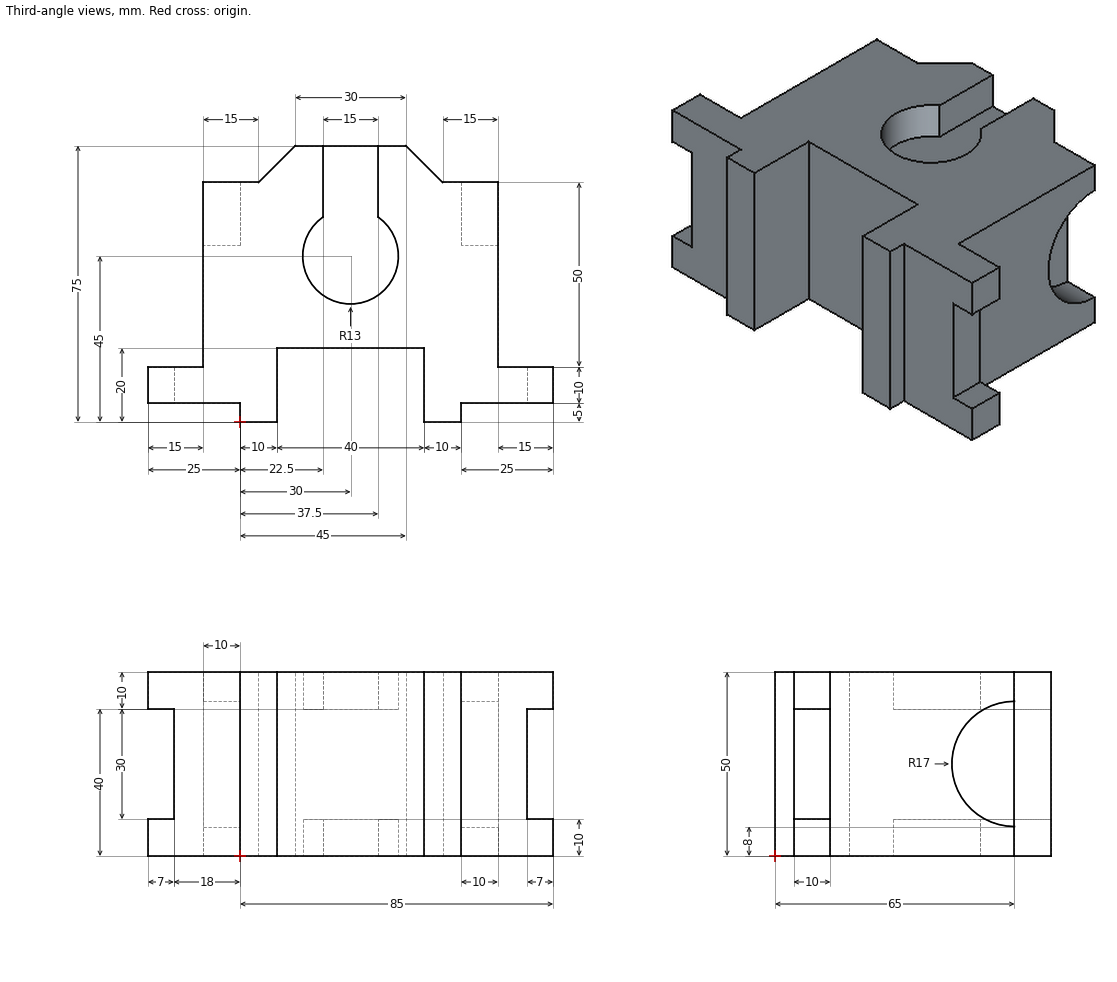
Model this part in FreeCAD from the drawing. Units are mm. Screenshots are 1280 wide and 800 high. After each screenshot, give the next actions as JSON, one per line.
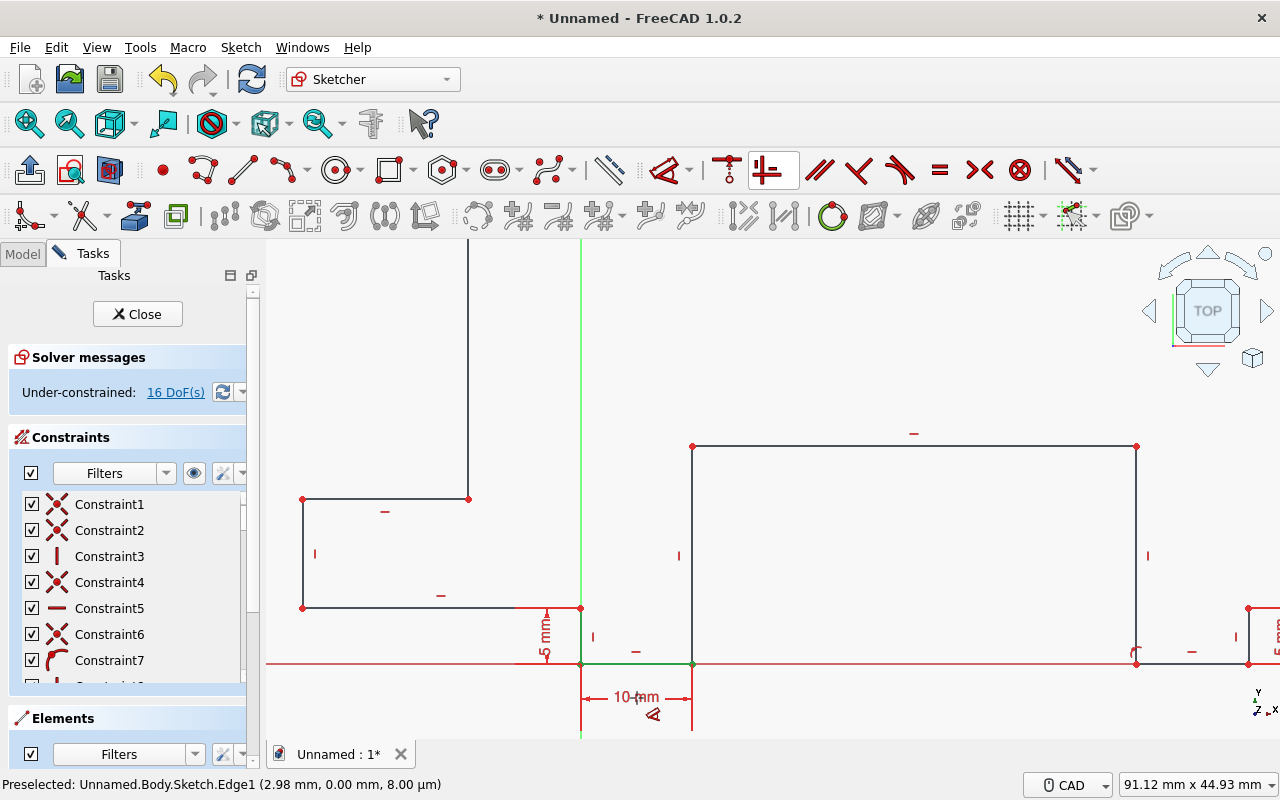
{"action": "left_click", "coordinate": [692, 599]}
{"action": "left_click", "coordinate": [658, 555]}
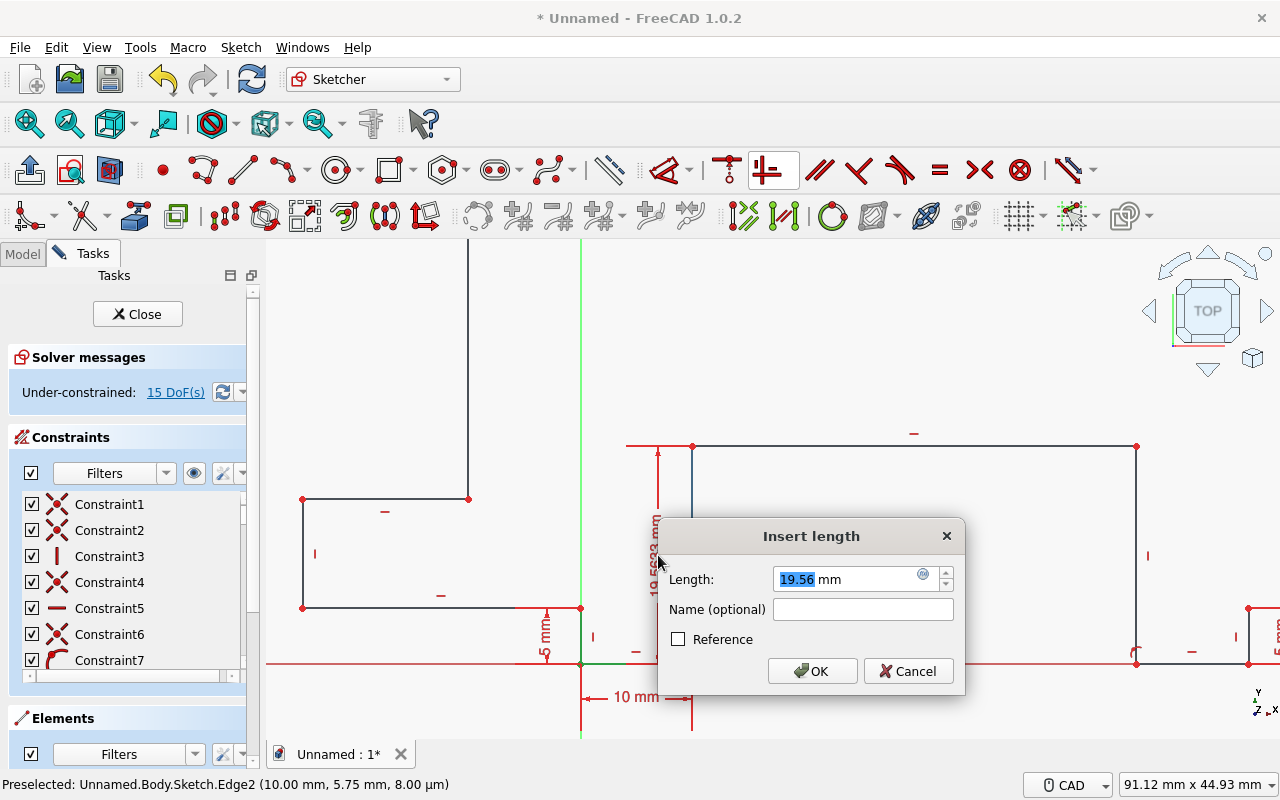
{"action": "type", "text": "20"}
{"action": "key", "text": "Return"}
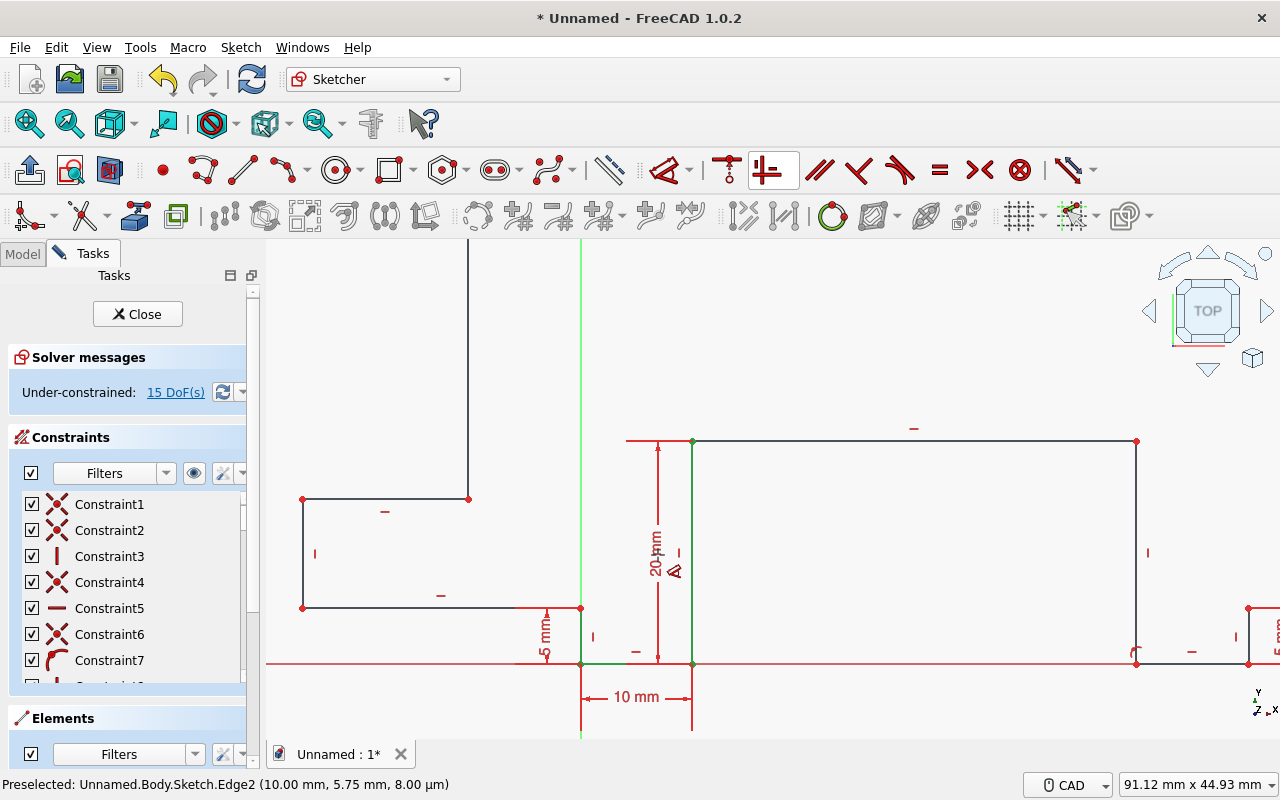
{"action": "left_click", "coordinate": [825, 441]}
{"action": "left_click", "coordinate": [904, 475]}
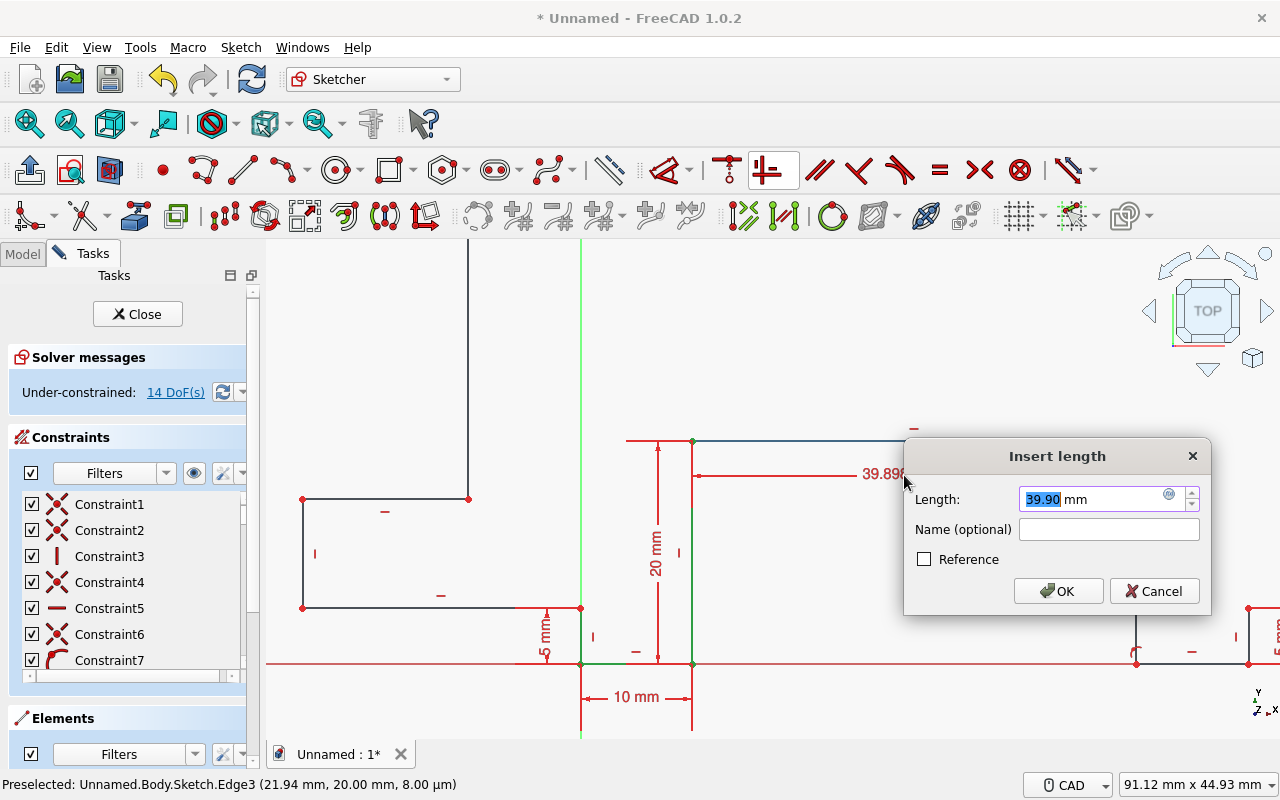
{"action": "type", "text": "40"}
{"action": "key", "text": "Return"}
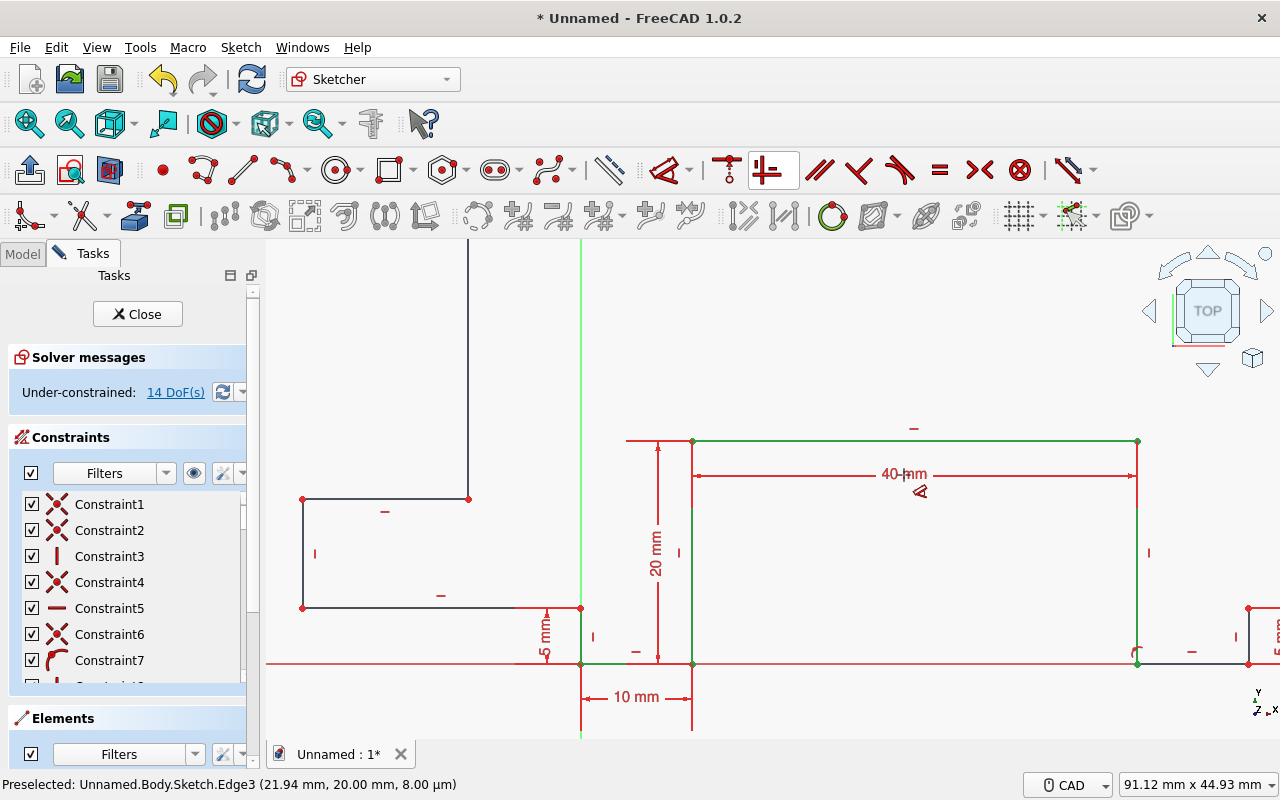
{"action": "scroll", "coordinate": [582, 630], "scroll_direction": "down", "scroll_amount": 5}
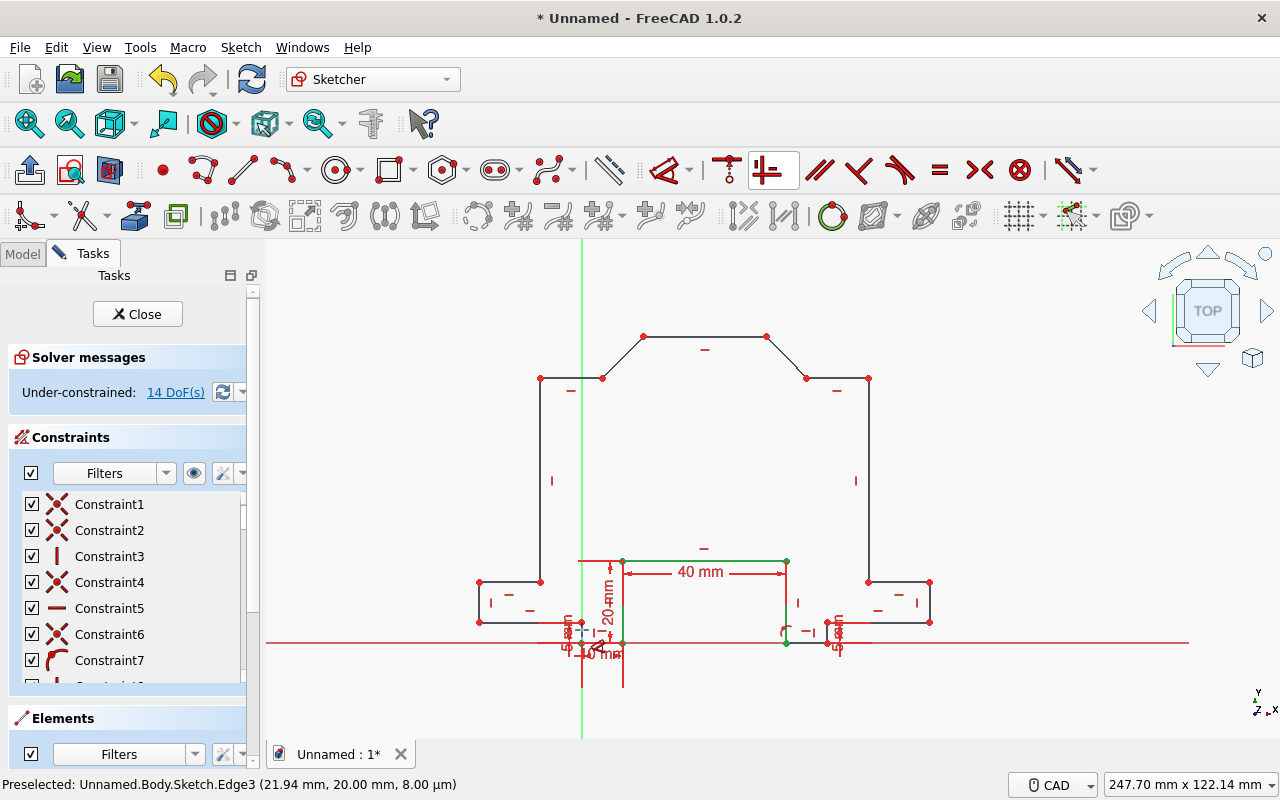
{"action": "left_click", "coordinate": [799, 643]}
{"action": "left_click", "coordinate": [807, 677]}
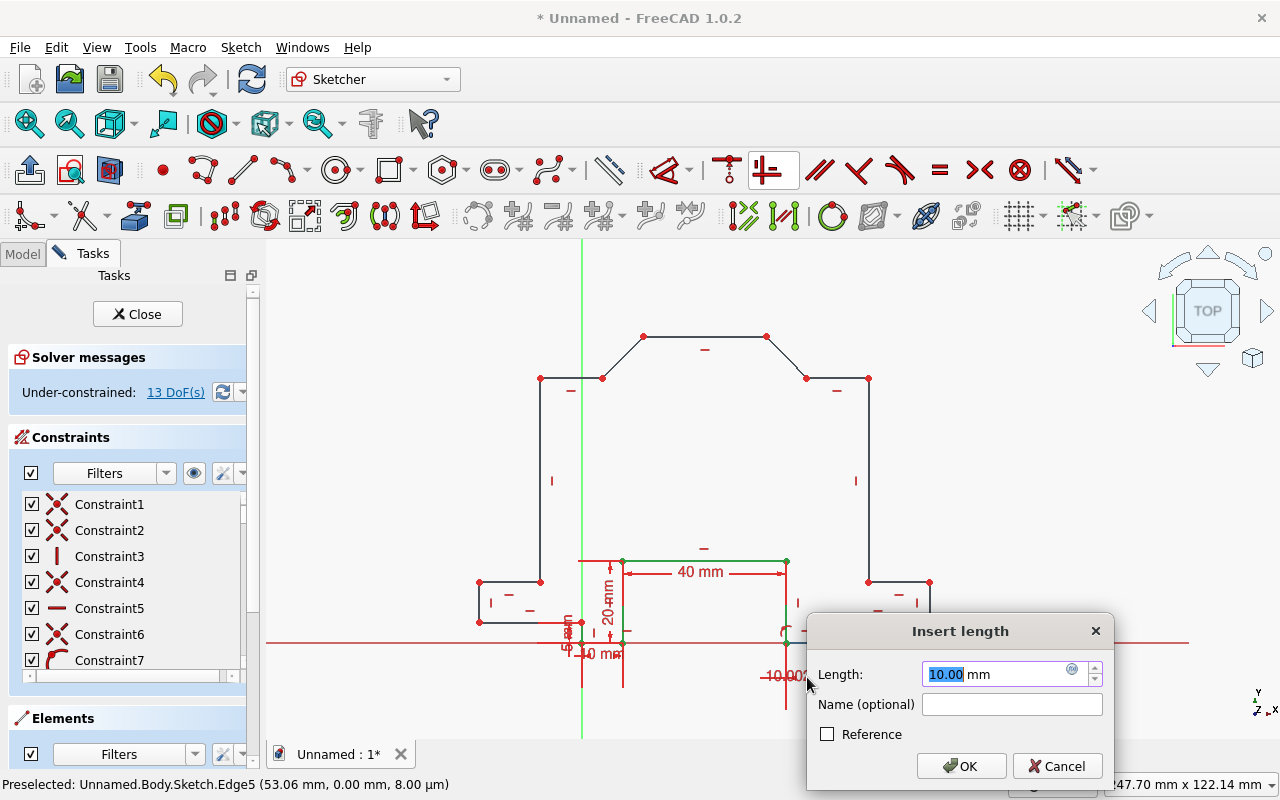
{"action": "type", "text": "10"}
{"action": "key", "text": "Return"}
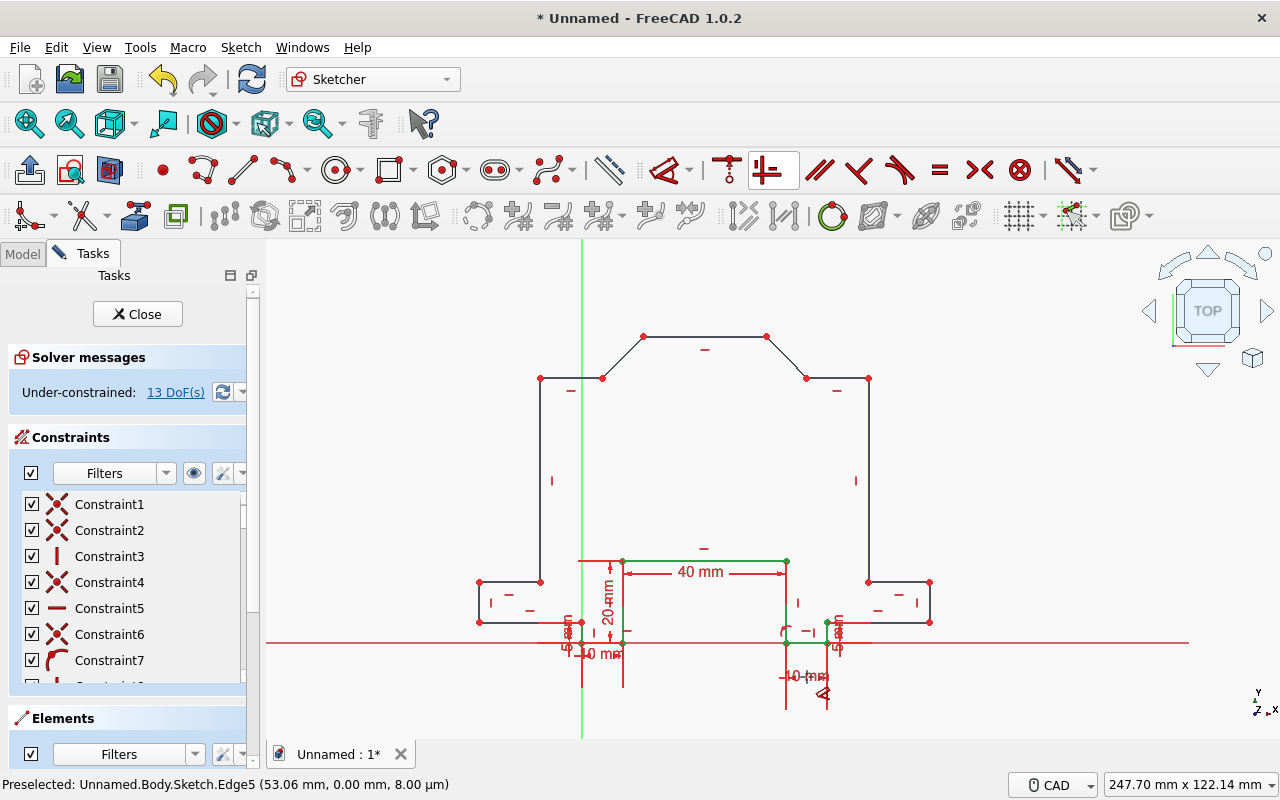
{"action": "left_click", "coordinate": [858, 623]}
{"action": "left_click", "coordinate": [878, 657]}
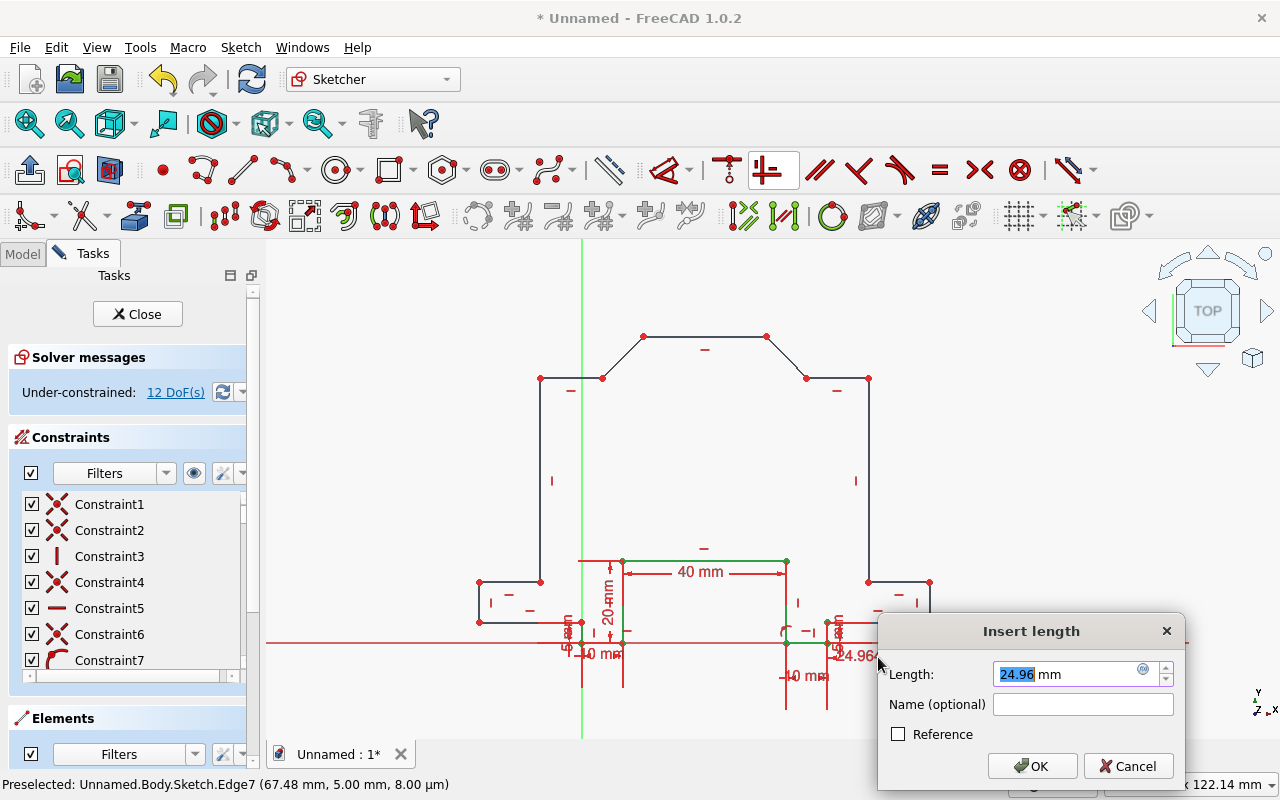
{"action": "type", "text": "25"}
{"action": "key", "text": "Return"}